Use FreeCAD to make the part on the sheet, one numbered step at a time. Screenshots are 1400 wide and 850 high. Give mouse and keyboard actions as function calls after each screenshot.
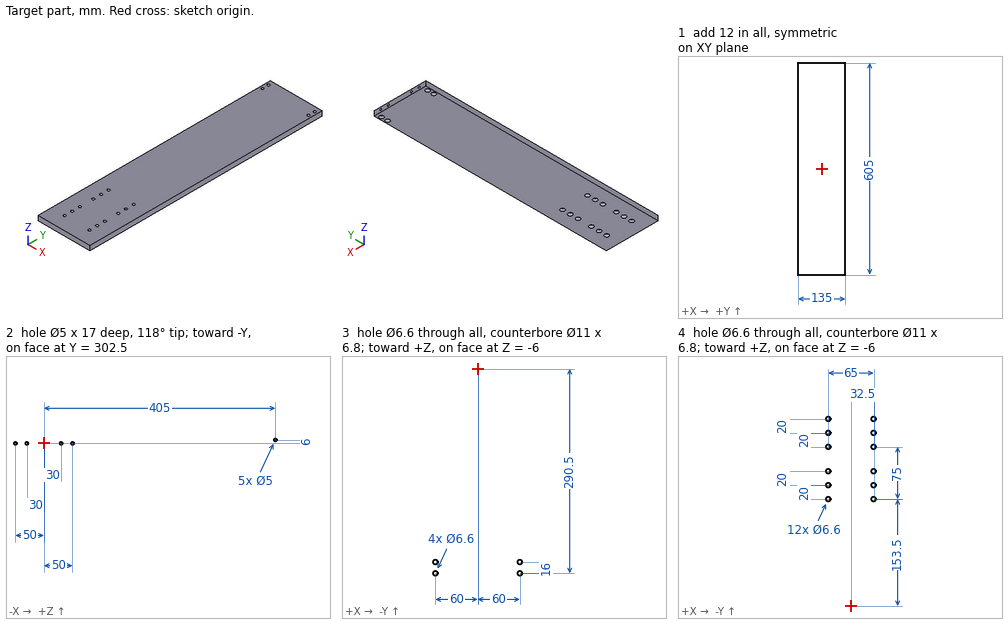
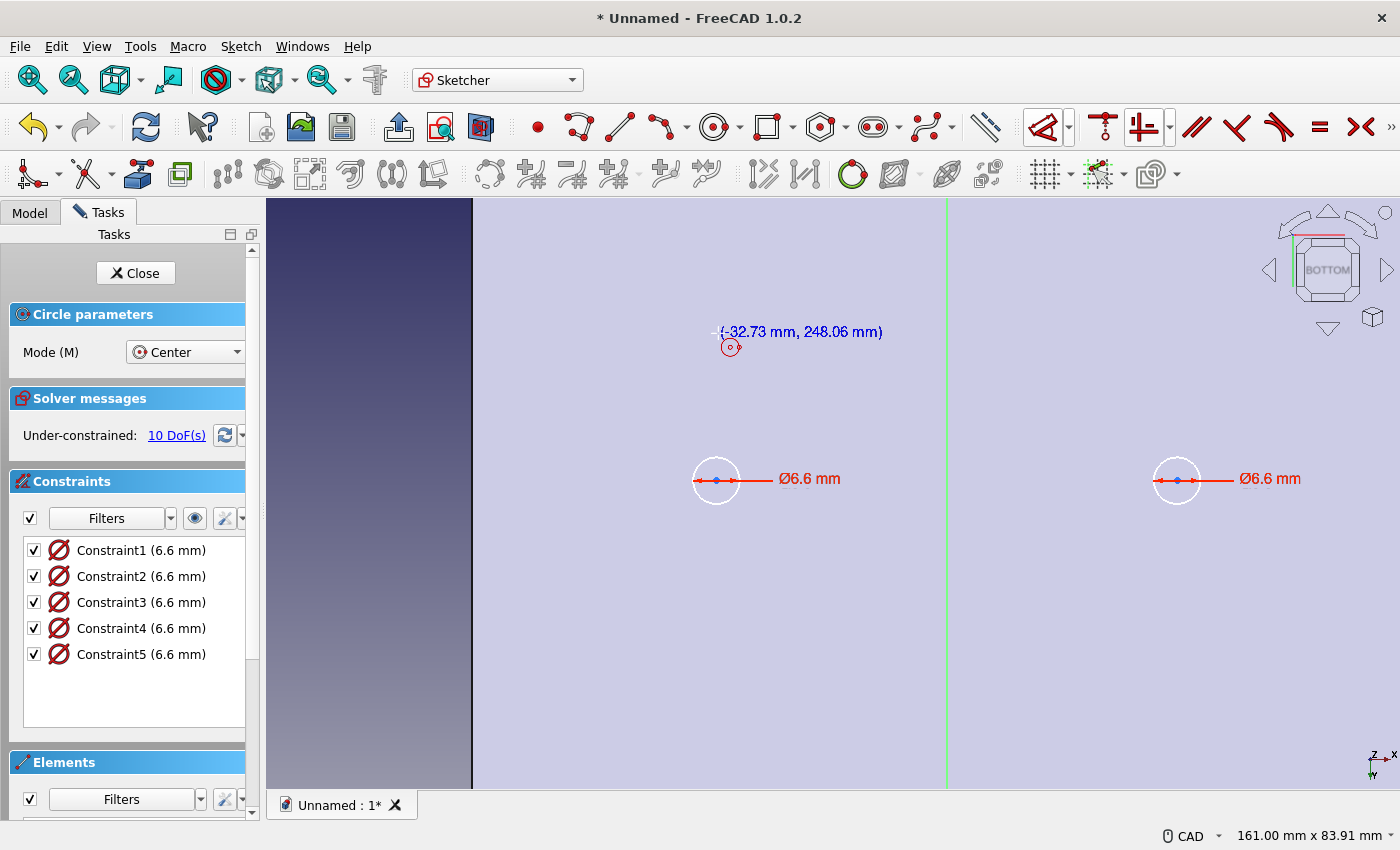
scroll(718, 333, down, 8)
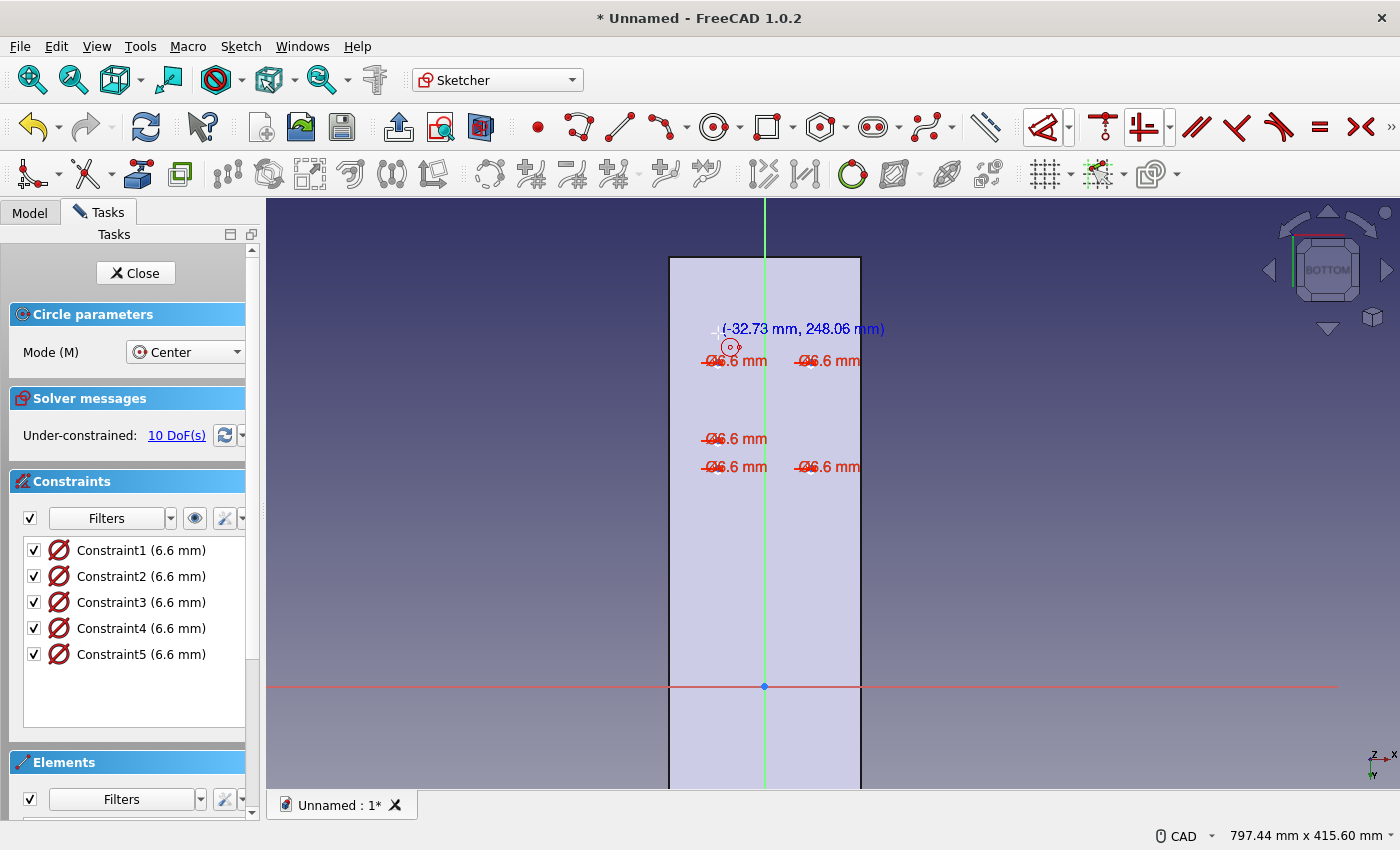
click(718, 333)
move(722, 330)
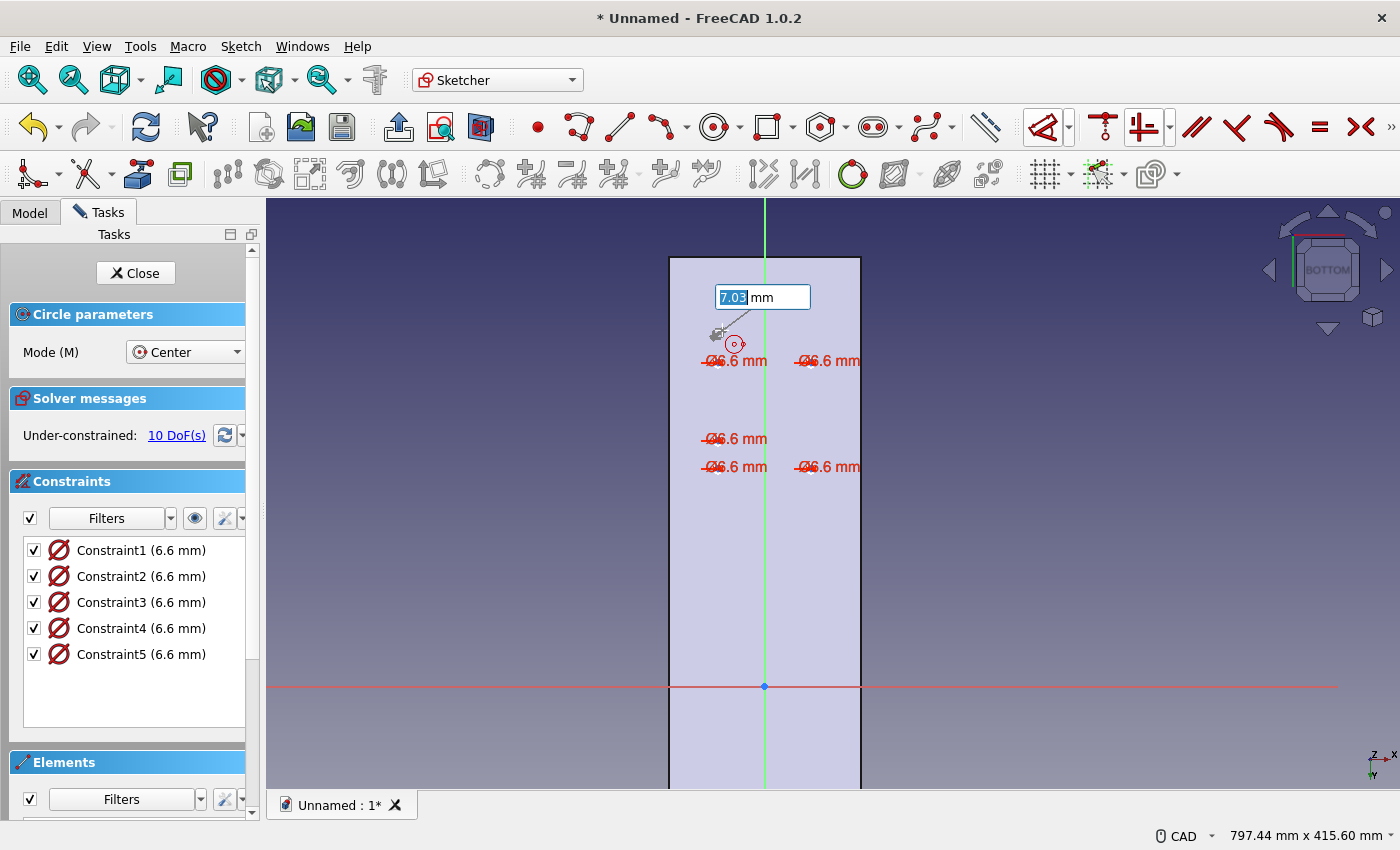
text(6.6)
key(Return)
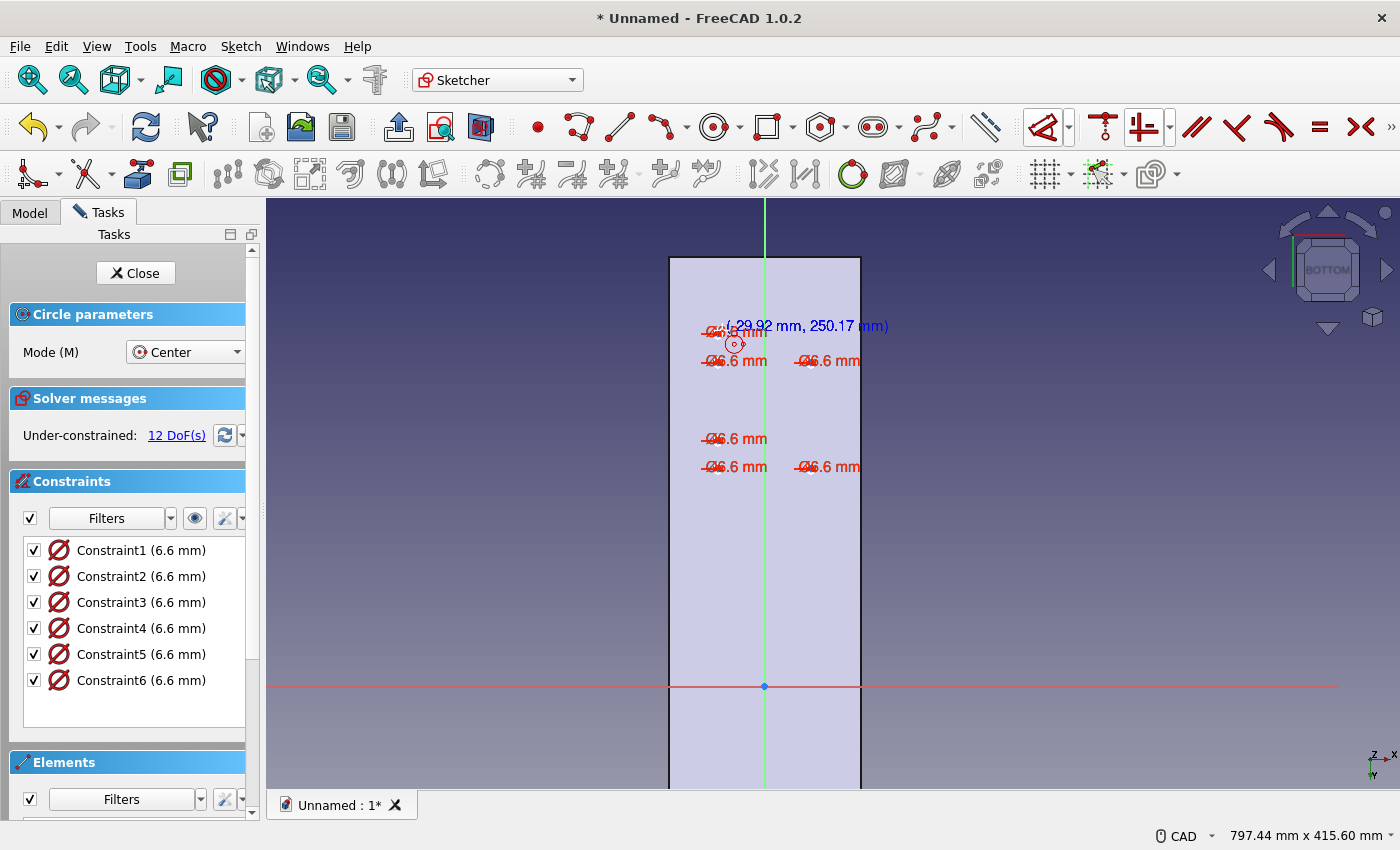
scroll(811, 333, up, 8)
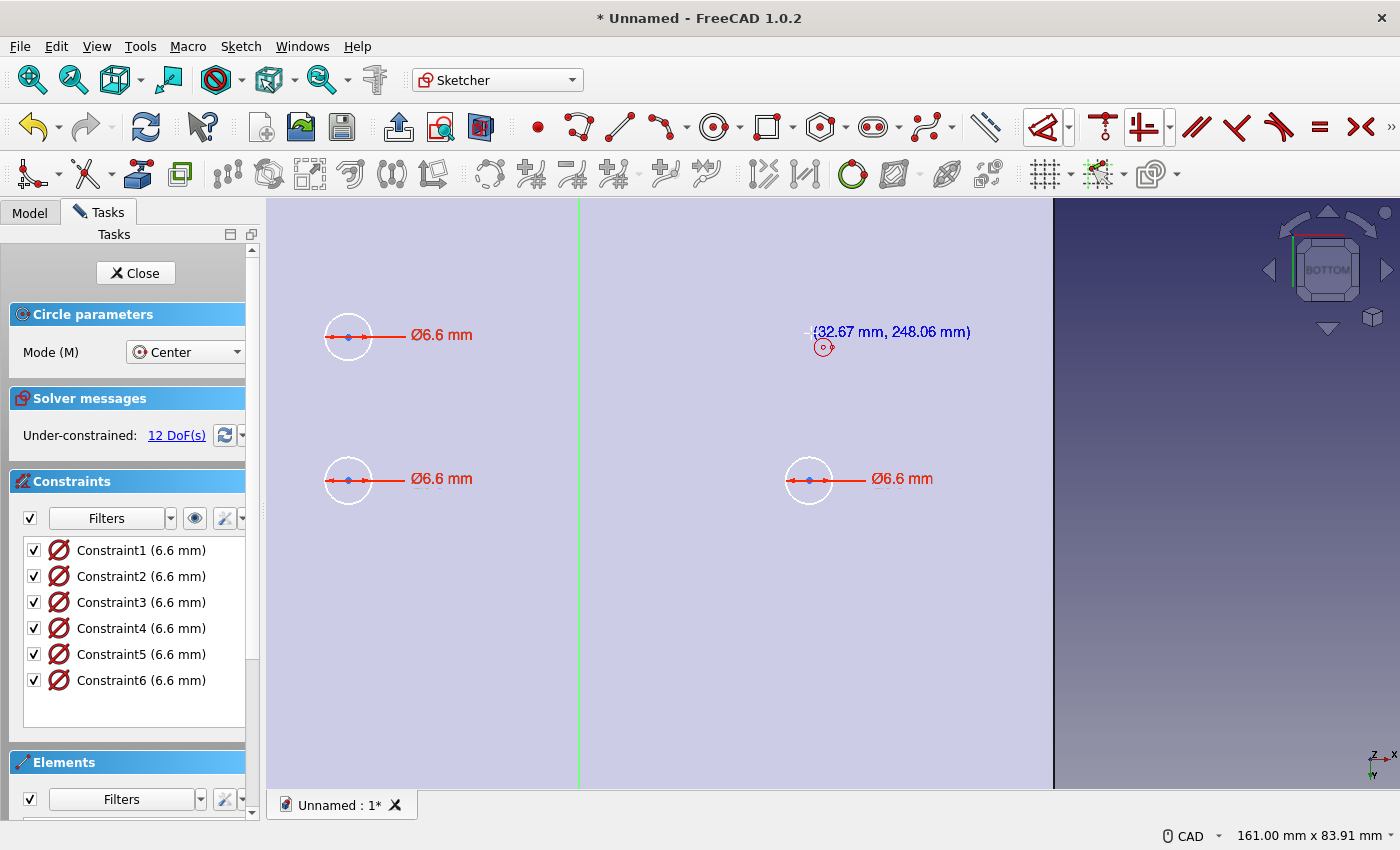
scroll(811, 333, down, 8)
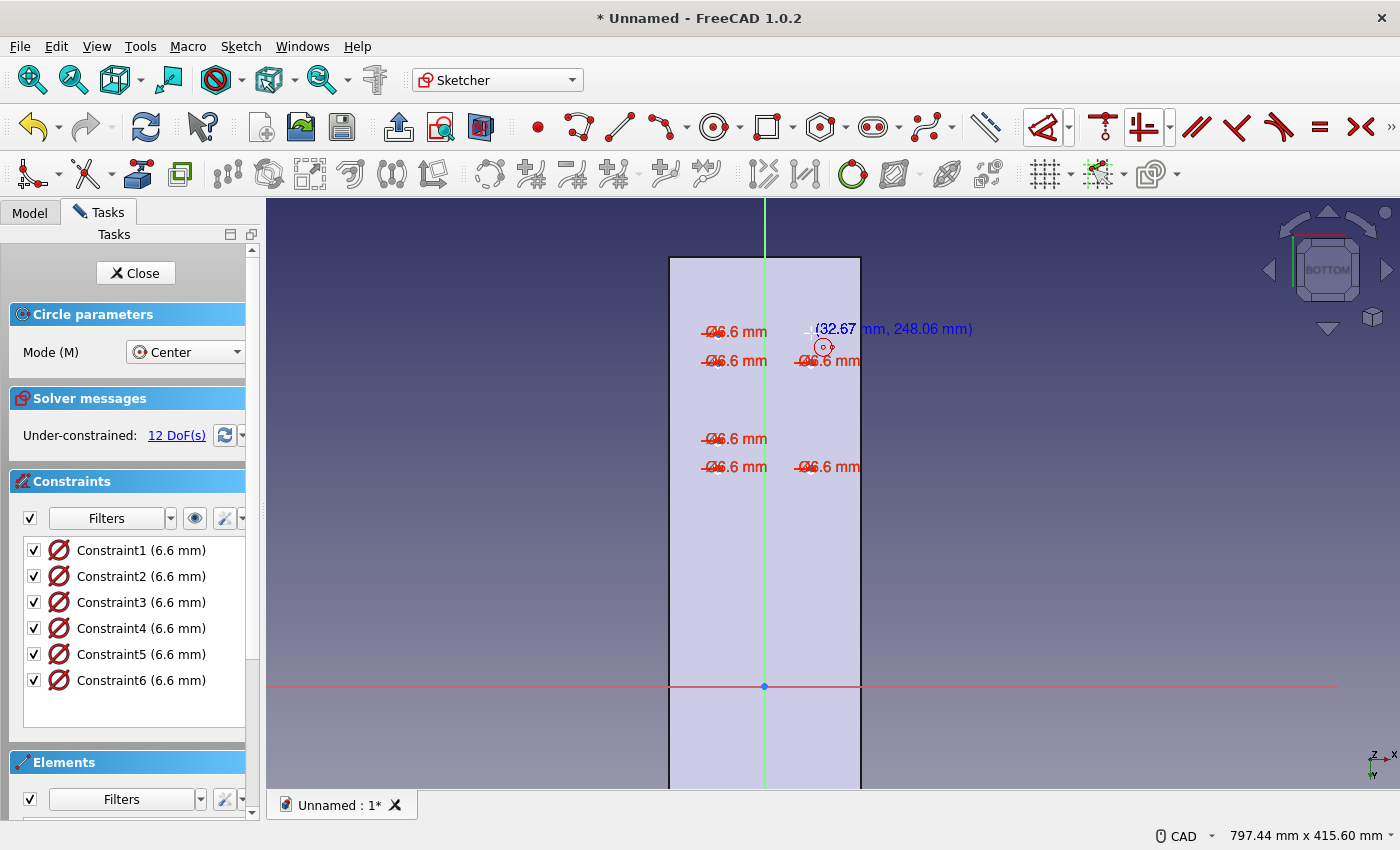
click(811, 333)
move(814, 330)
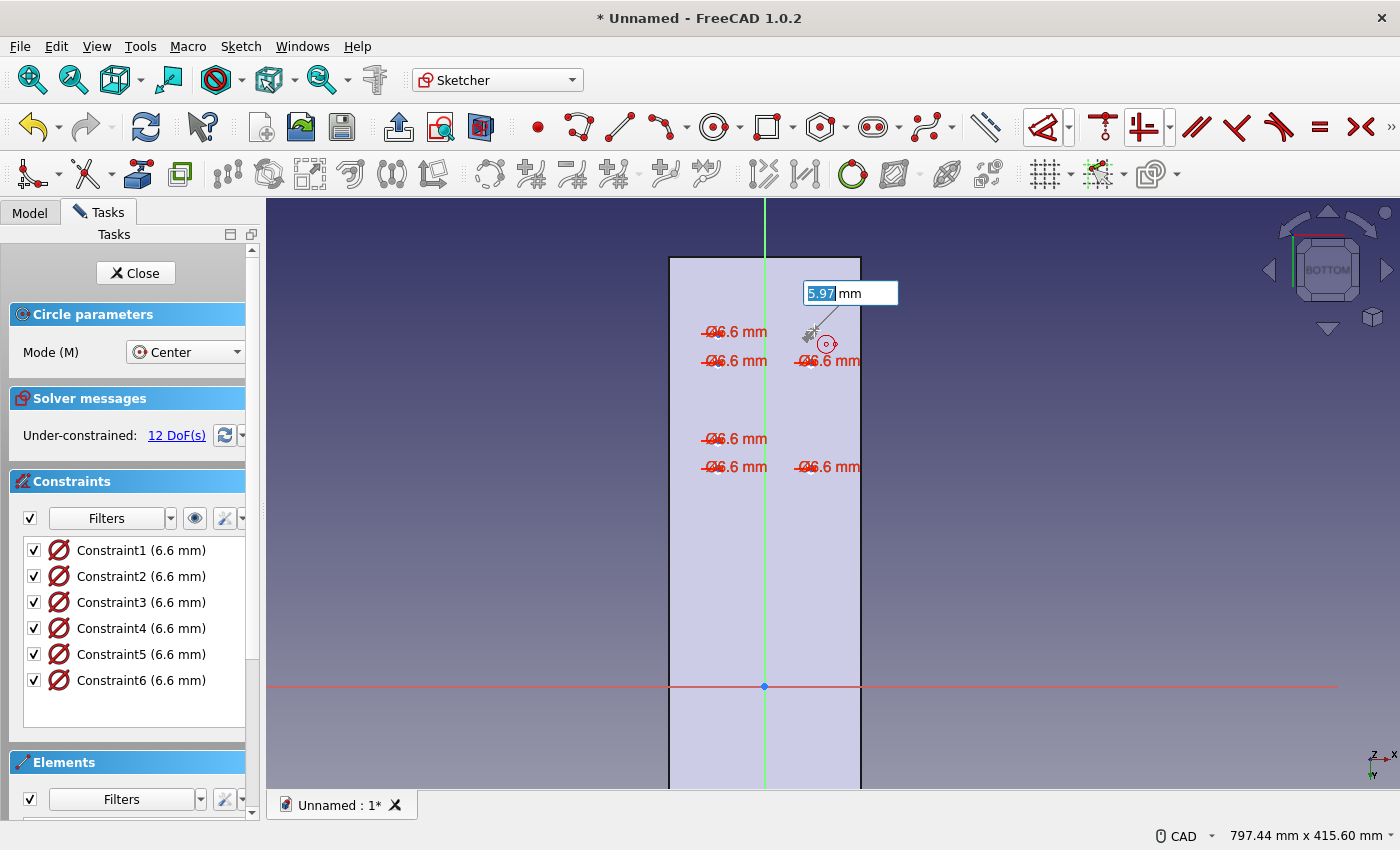
text(6.6)
key(Return)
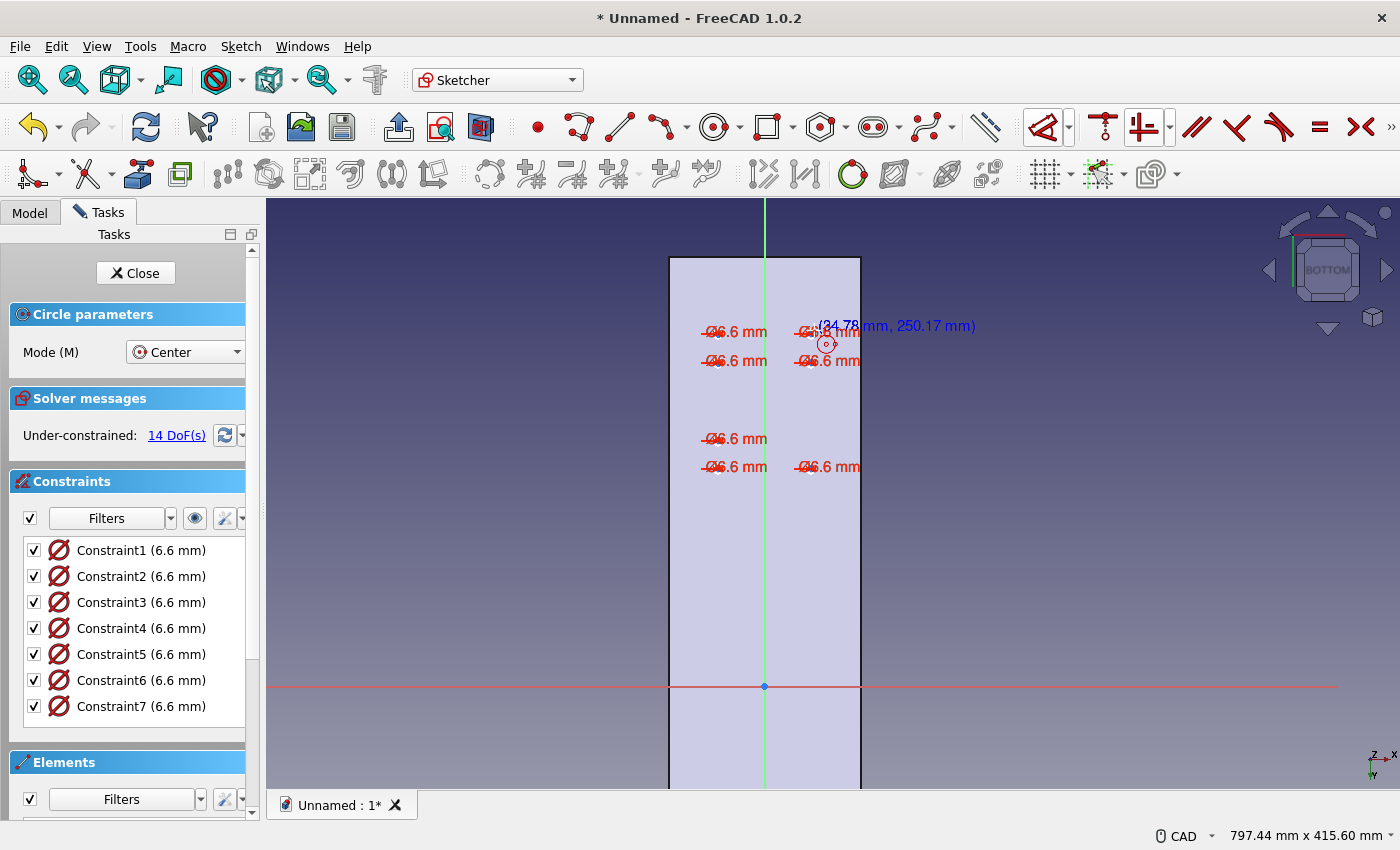
scroll(811, 440, up, 8)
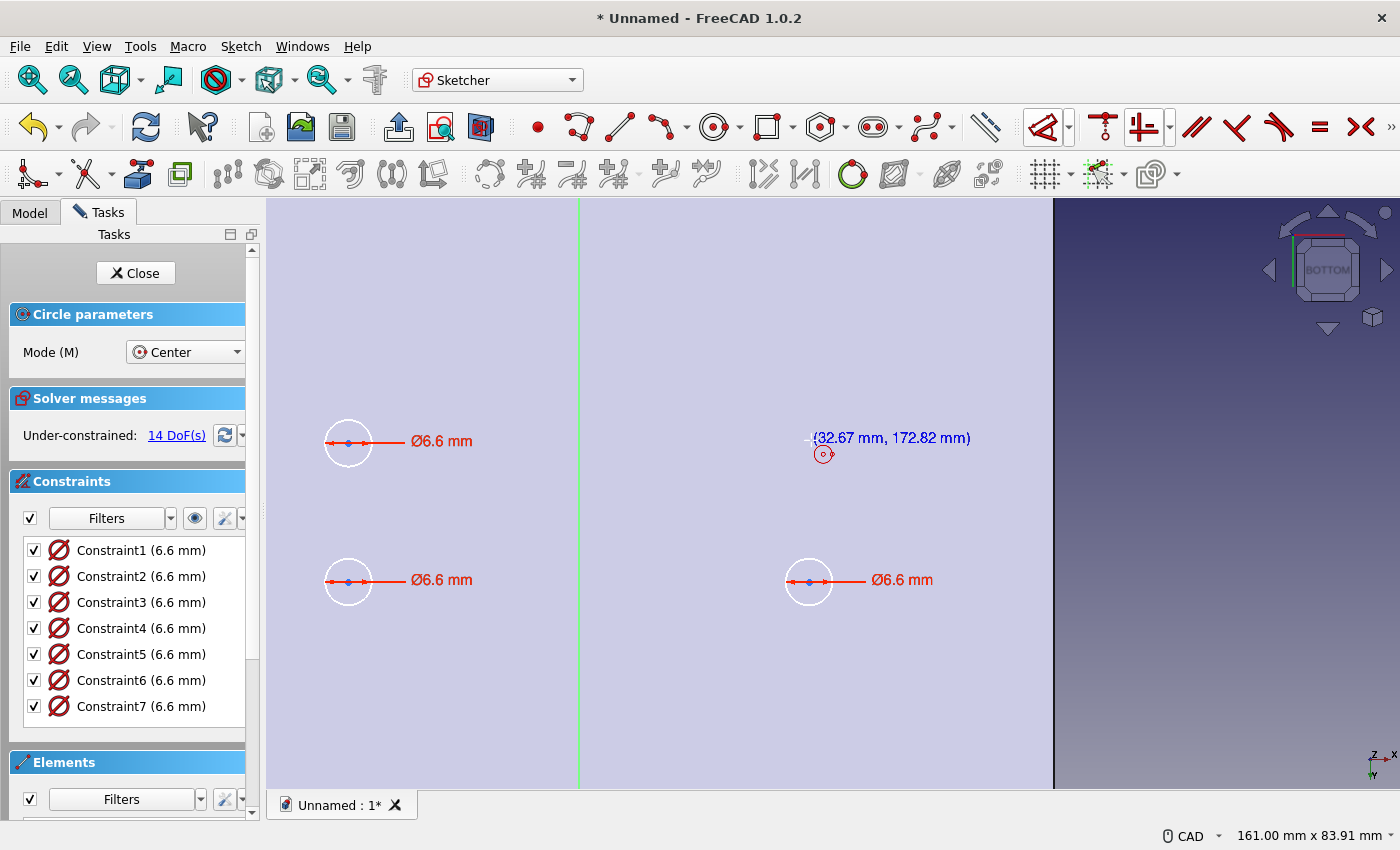
scroll(811, 440, down, 8)